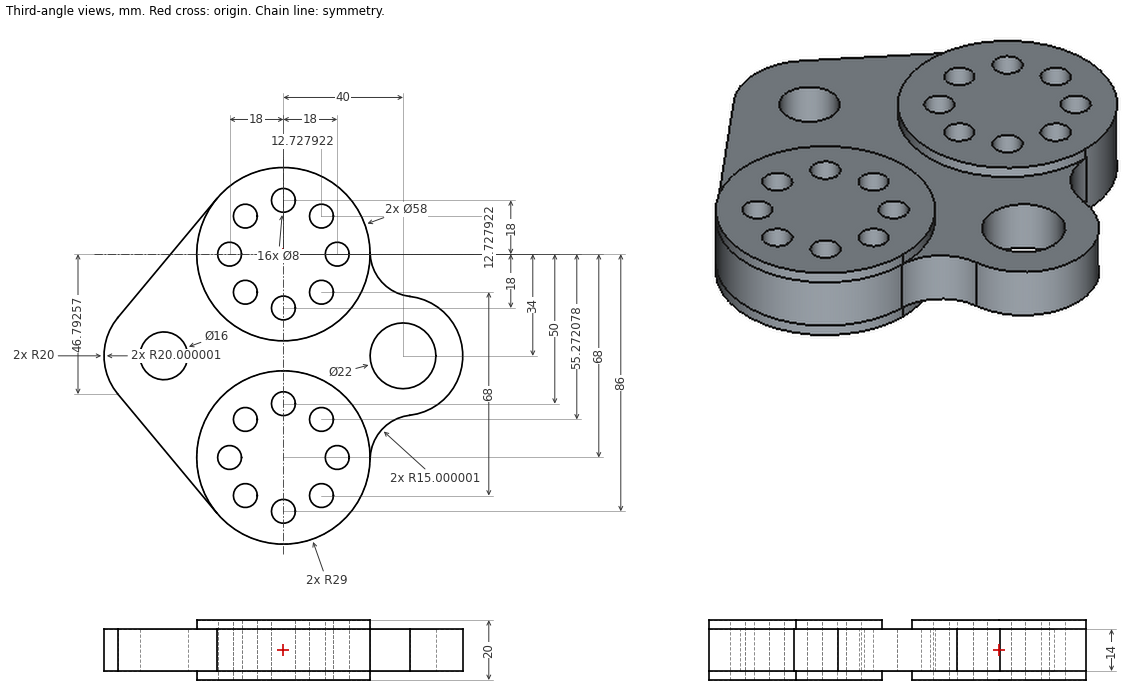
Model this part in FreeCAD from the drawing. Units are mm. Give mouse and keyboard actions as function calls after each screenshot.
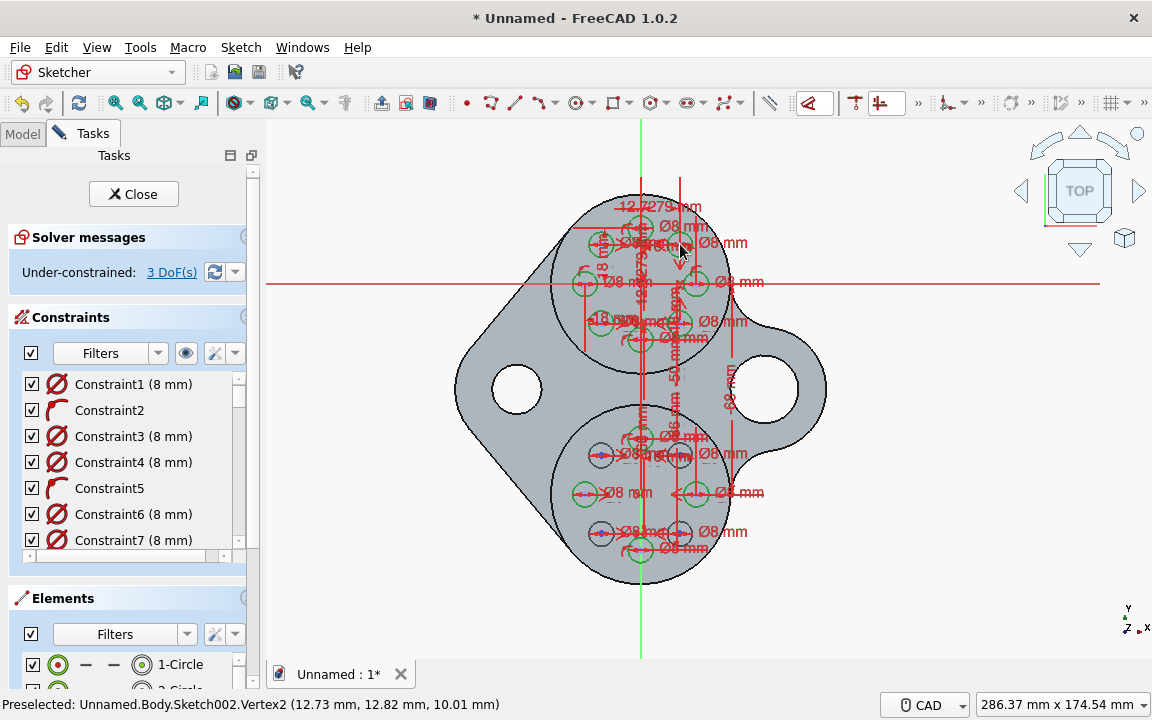
click(680, 456)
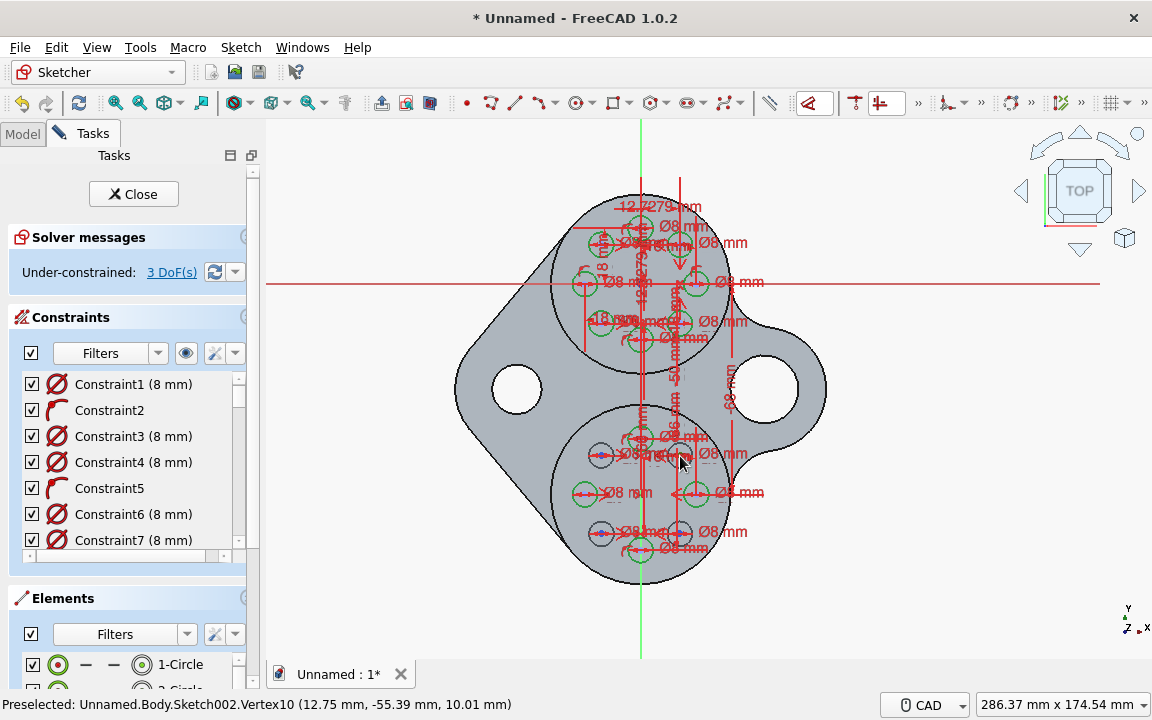
key(l)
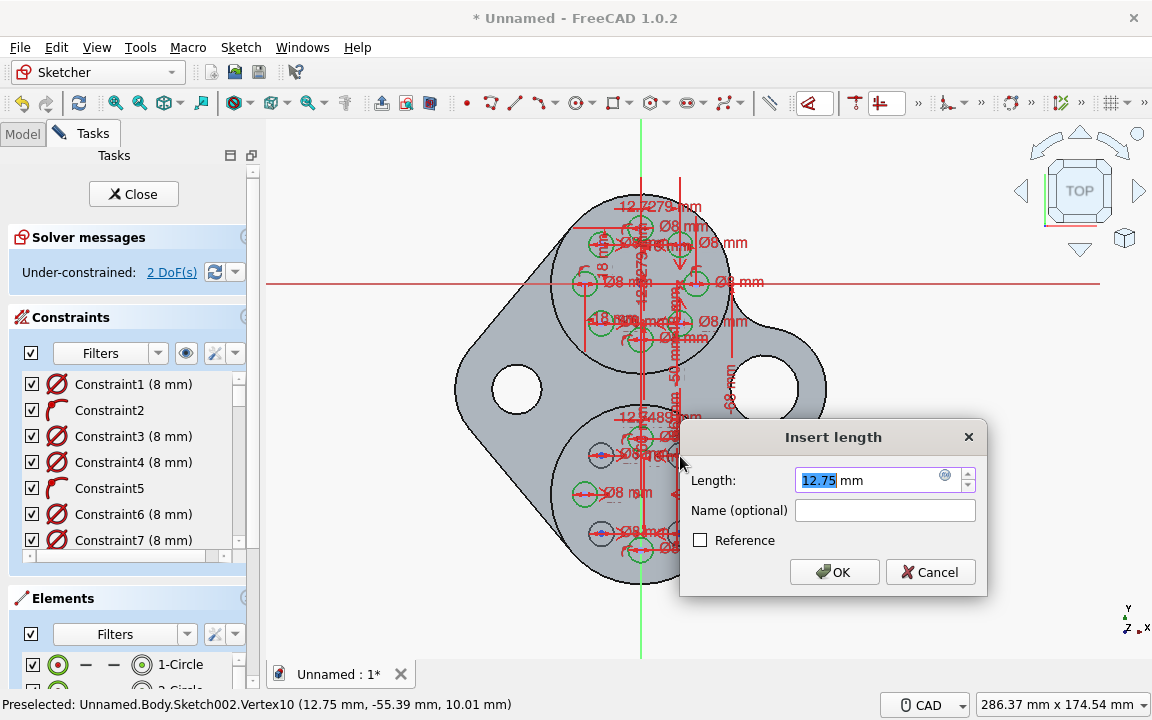
text(12.727922)
key(Return)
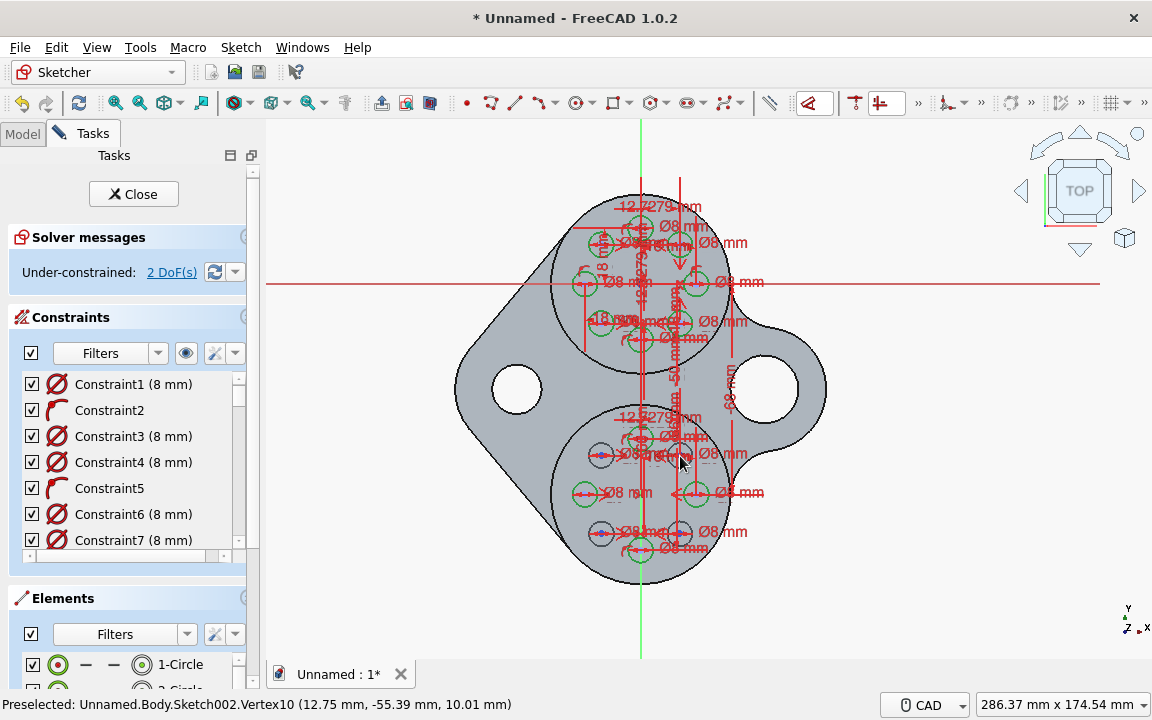
click(680, 456)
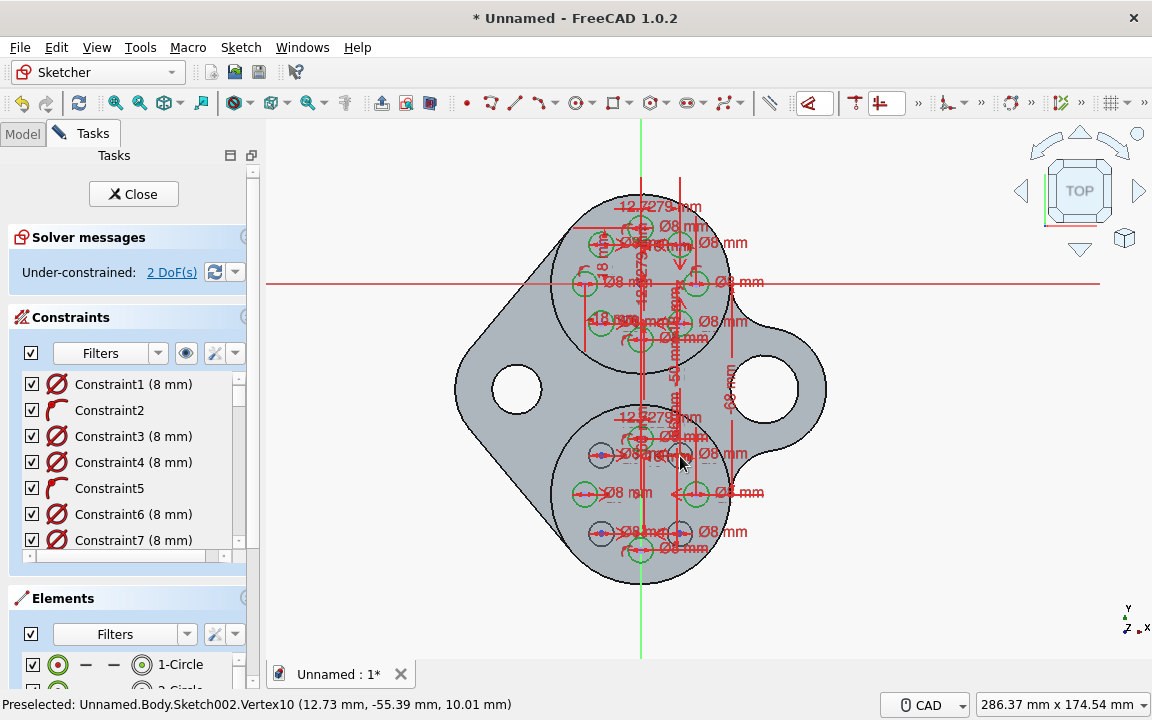
key(i)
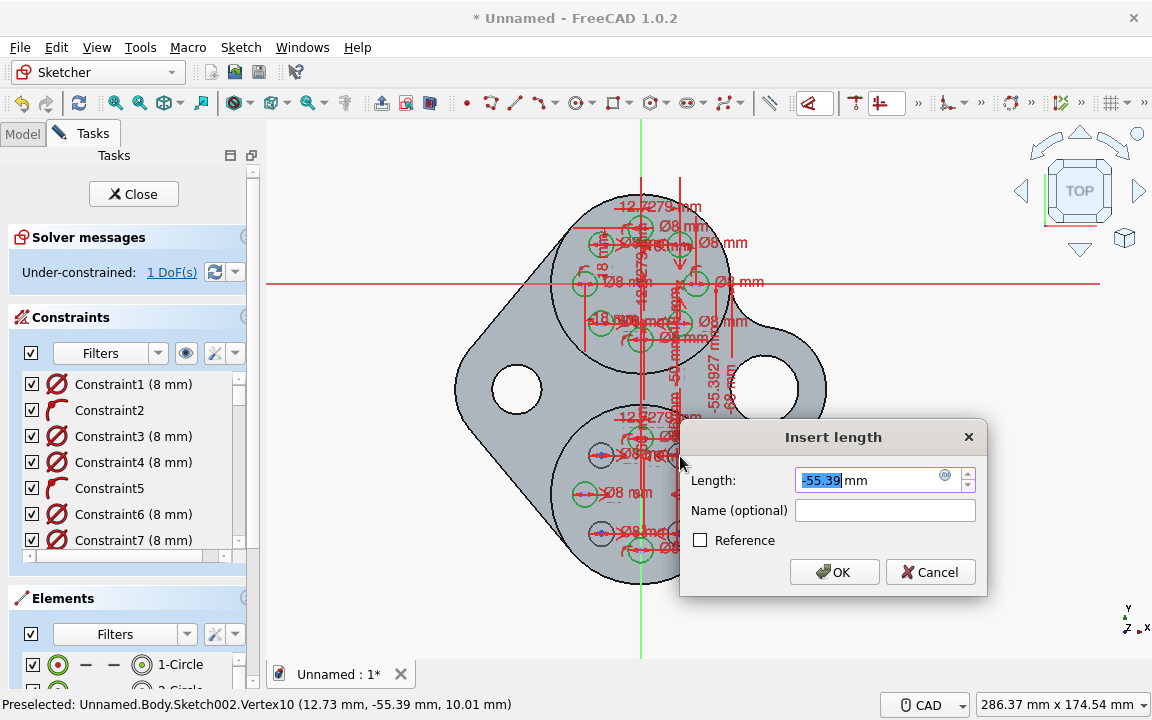
text(-55.272078)
key(Return)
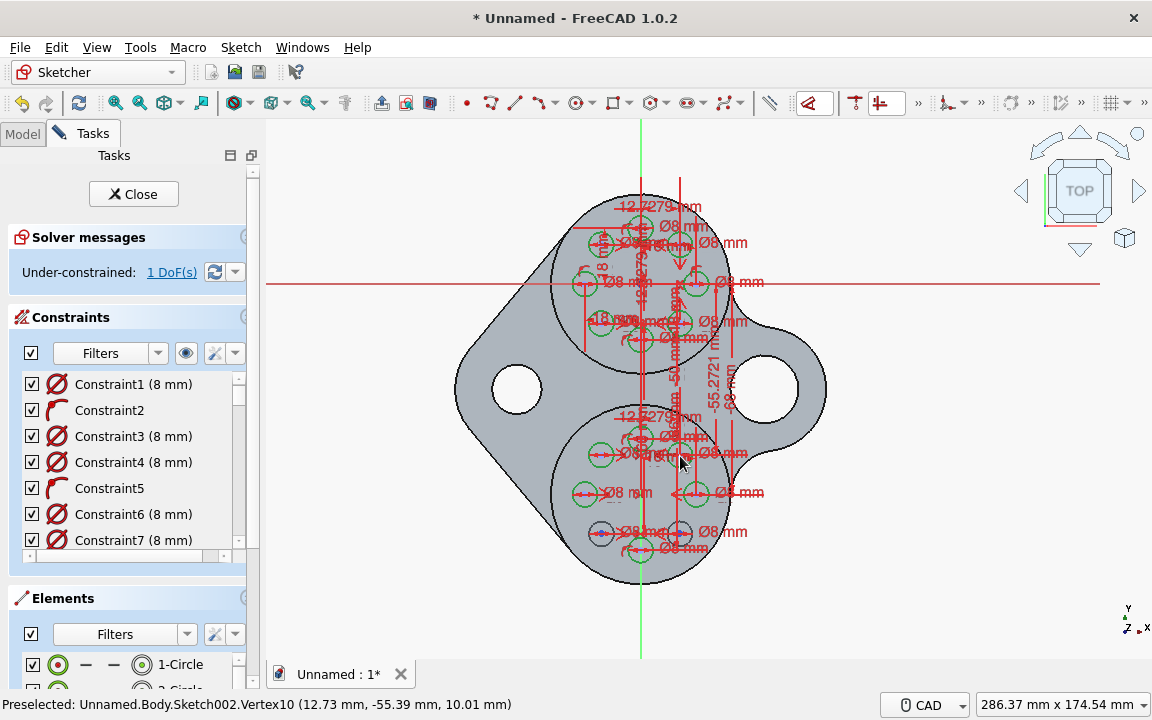
click(680, 534)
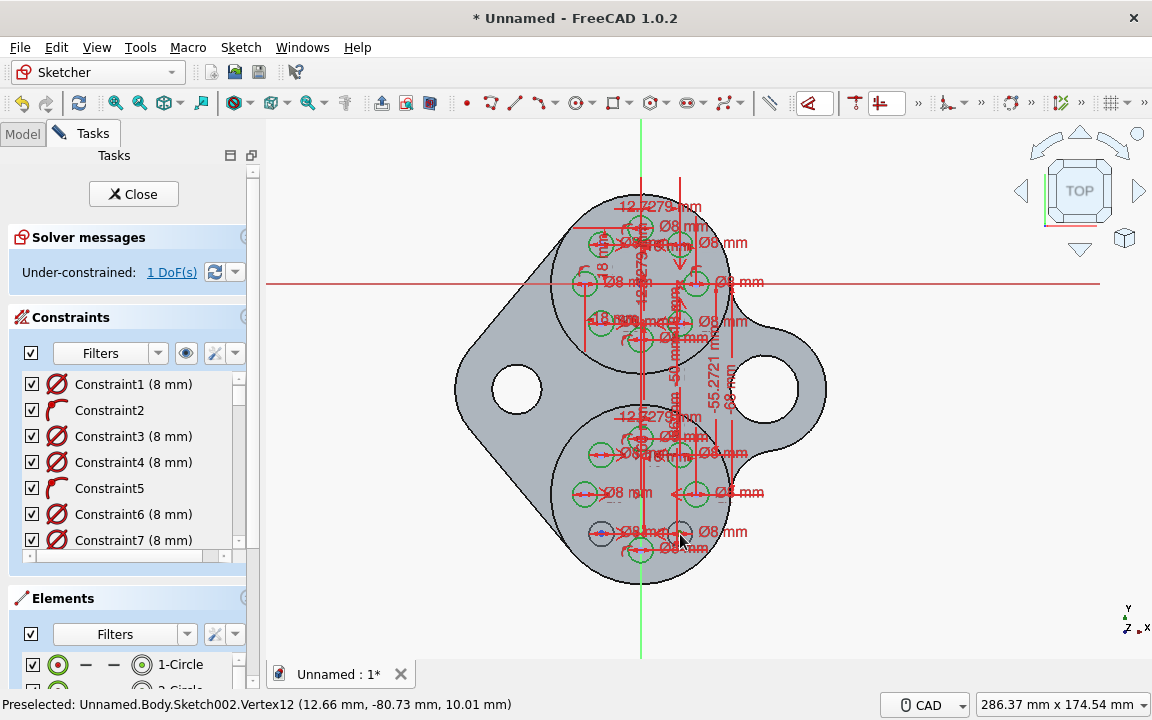
key(l)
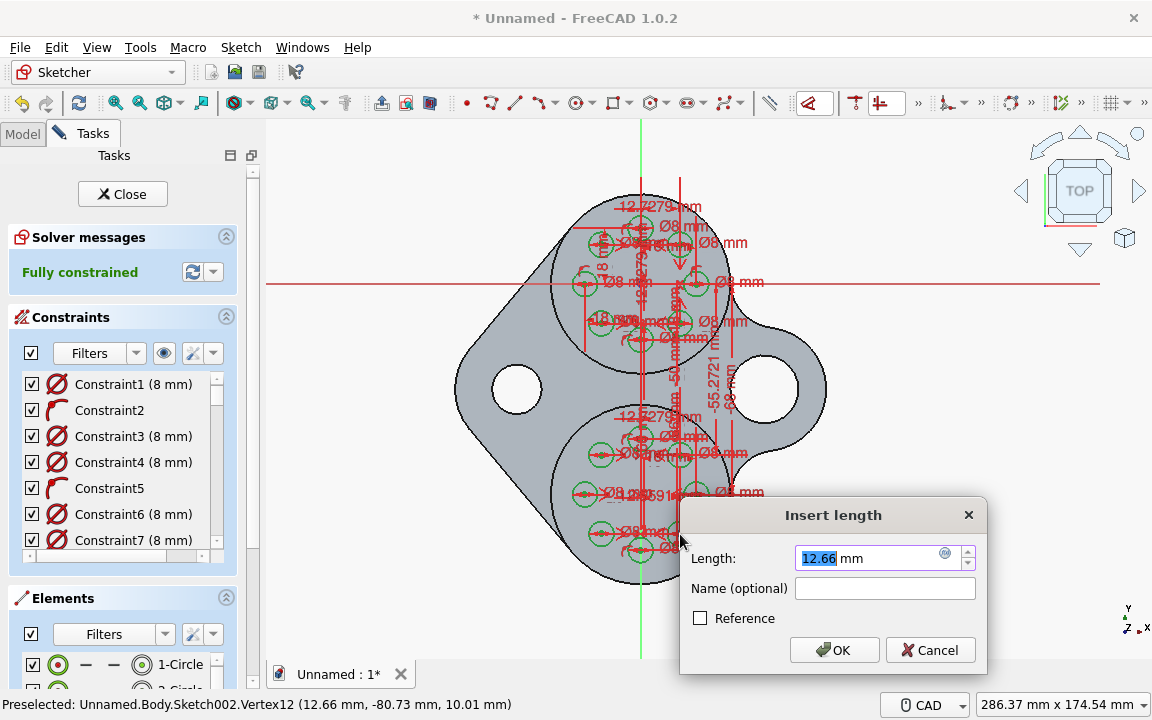
text(12.727922)
key(Return)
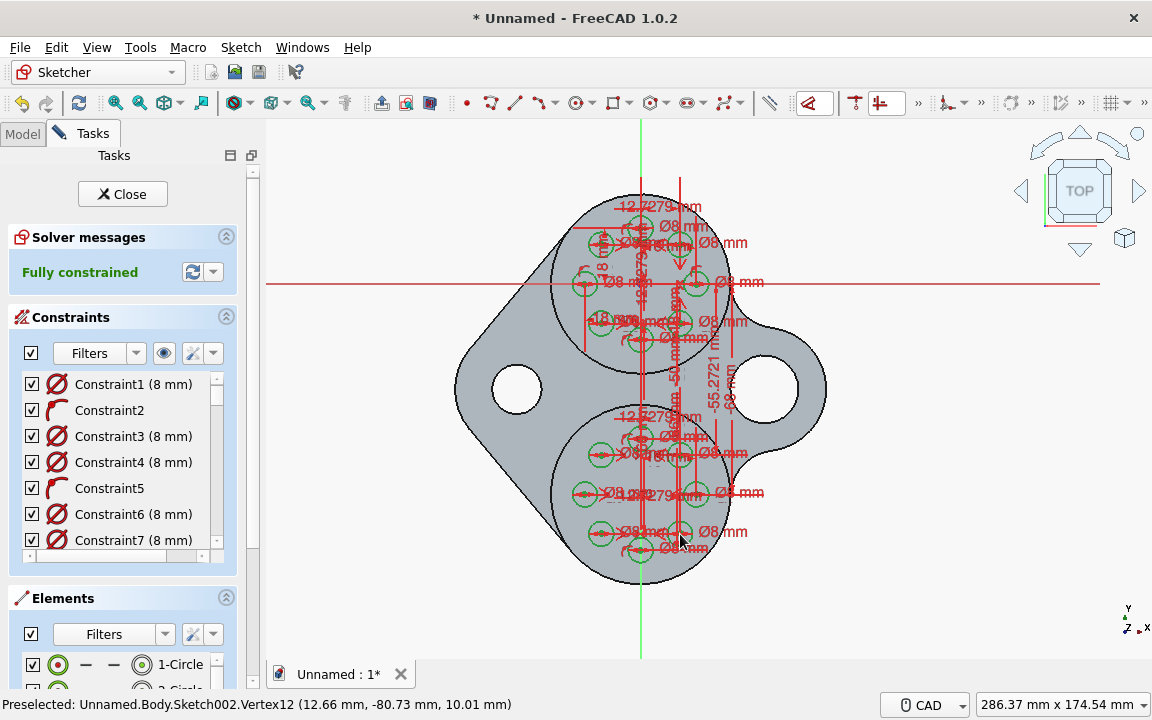
click(123, 194)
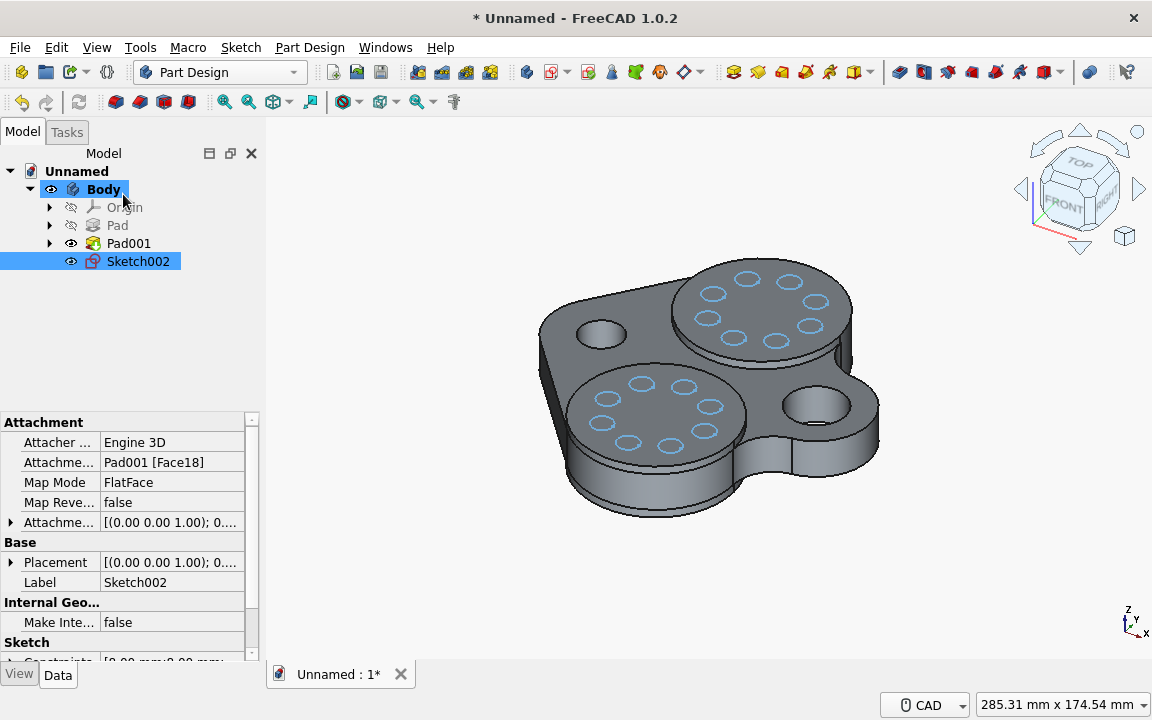
click(900, 72)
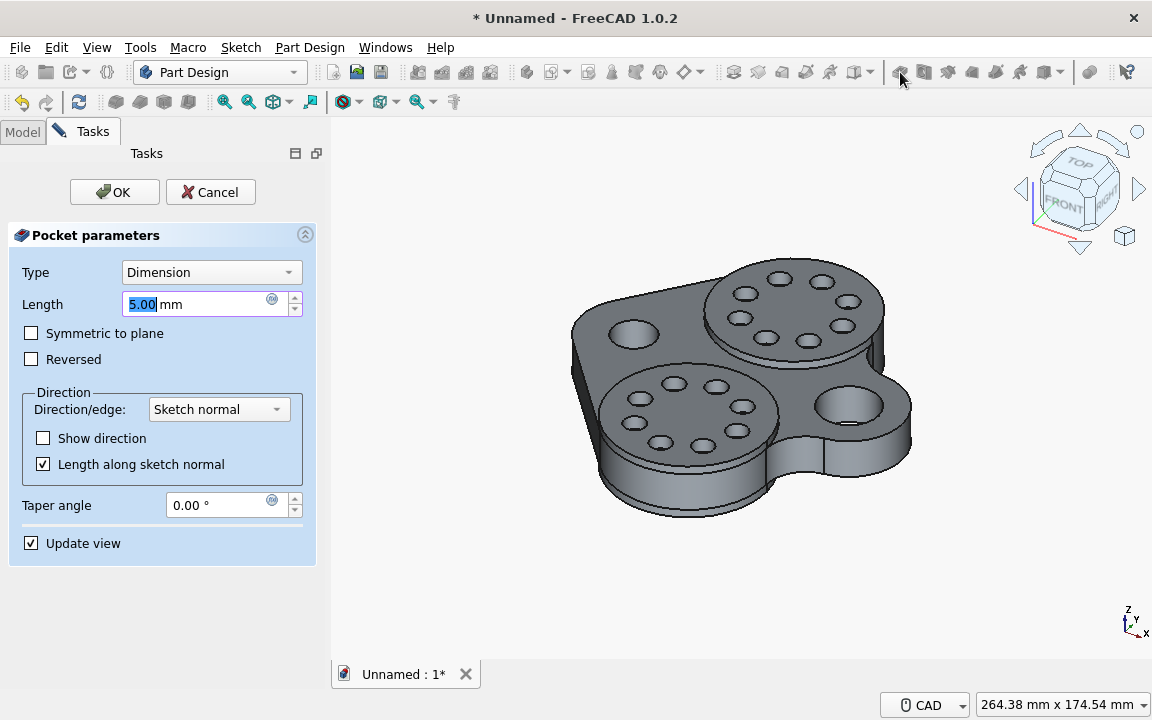
click(212, 272)